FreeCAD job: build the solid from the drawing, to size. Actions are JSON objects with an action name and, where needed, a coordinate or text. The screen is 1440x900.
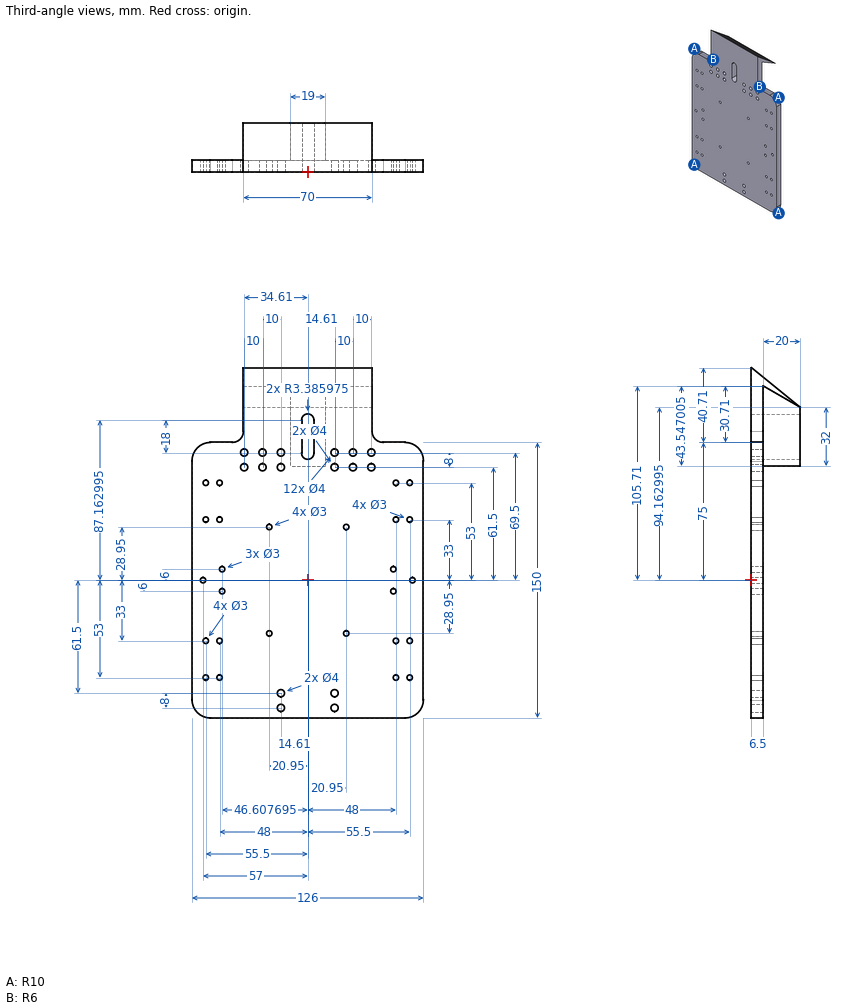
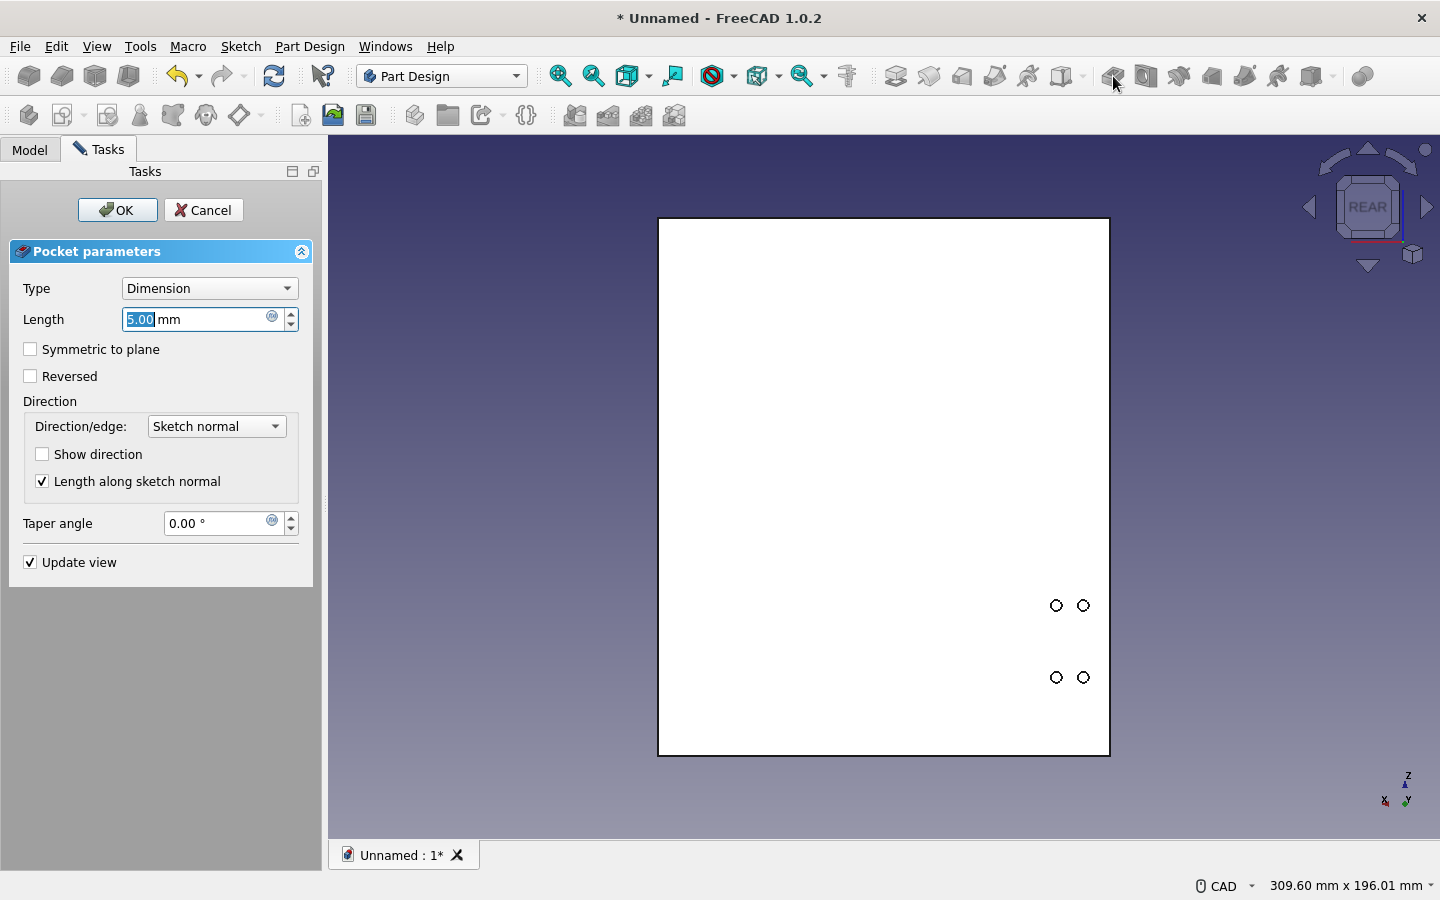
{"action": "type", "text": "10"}
{"action": "key", "text": "Tab"}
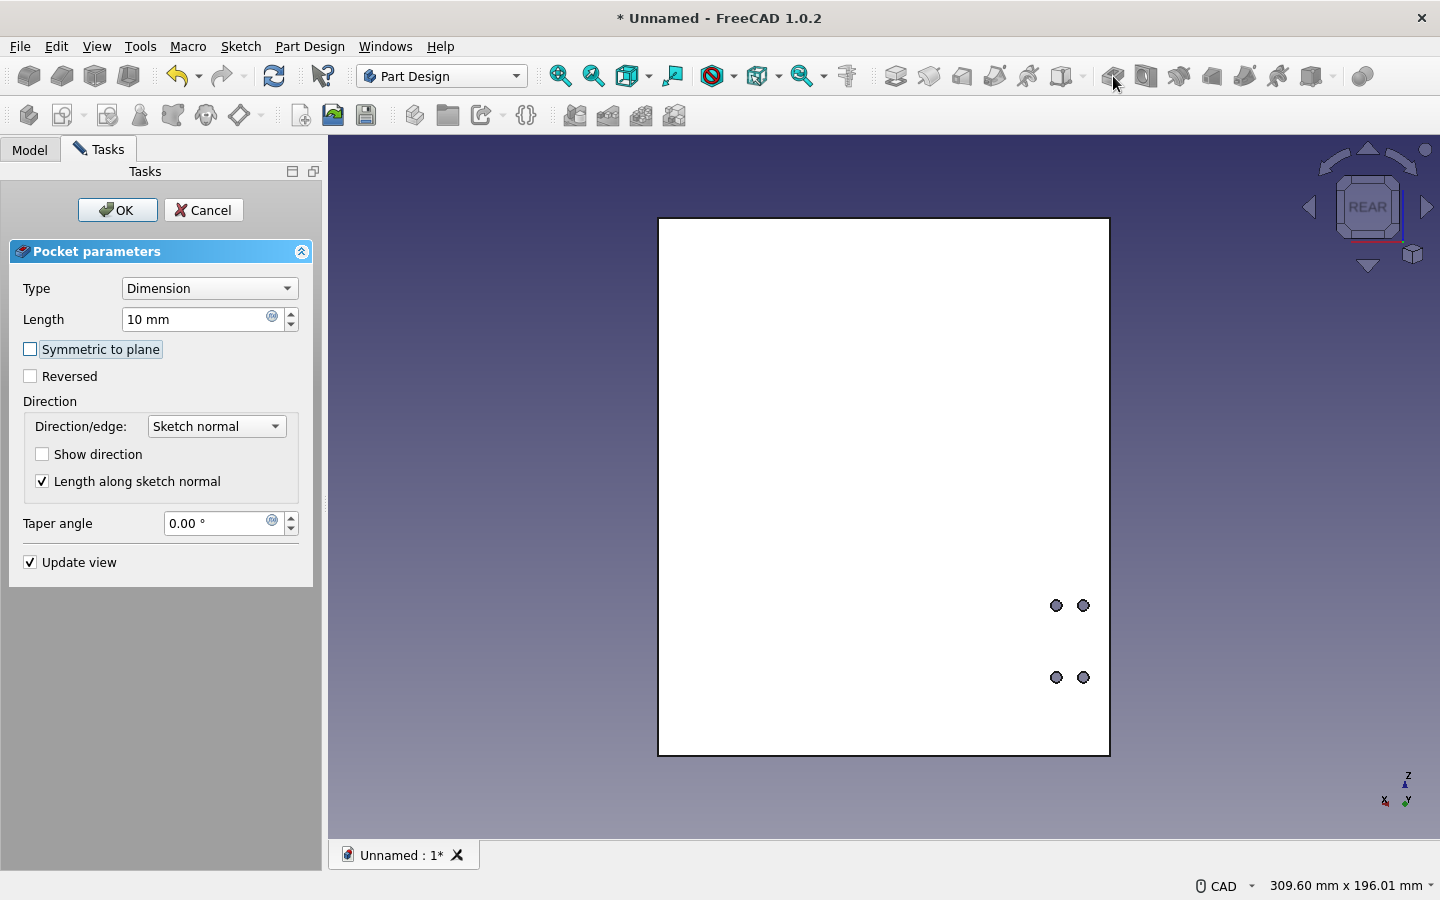
{"action": "left_click", "coordinate": [118, 210]}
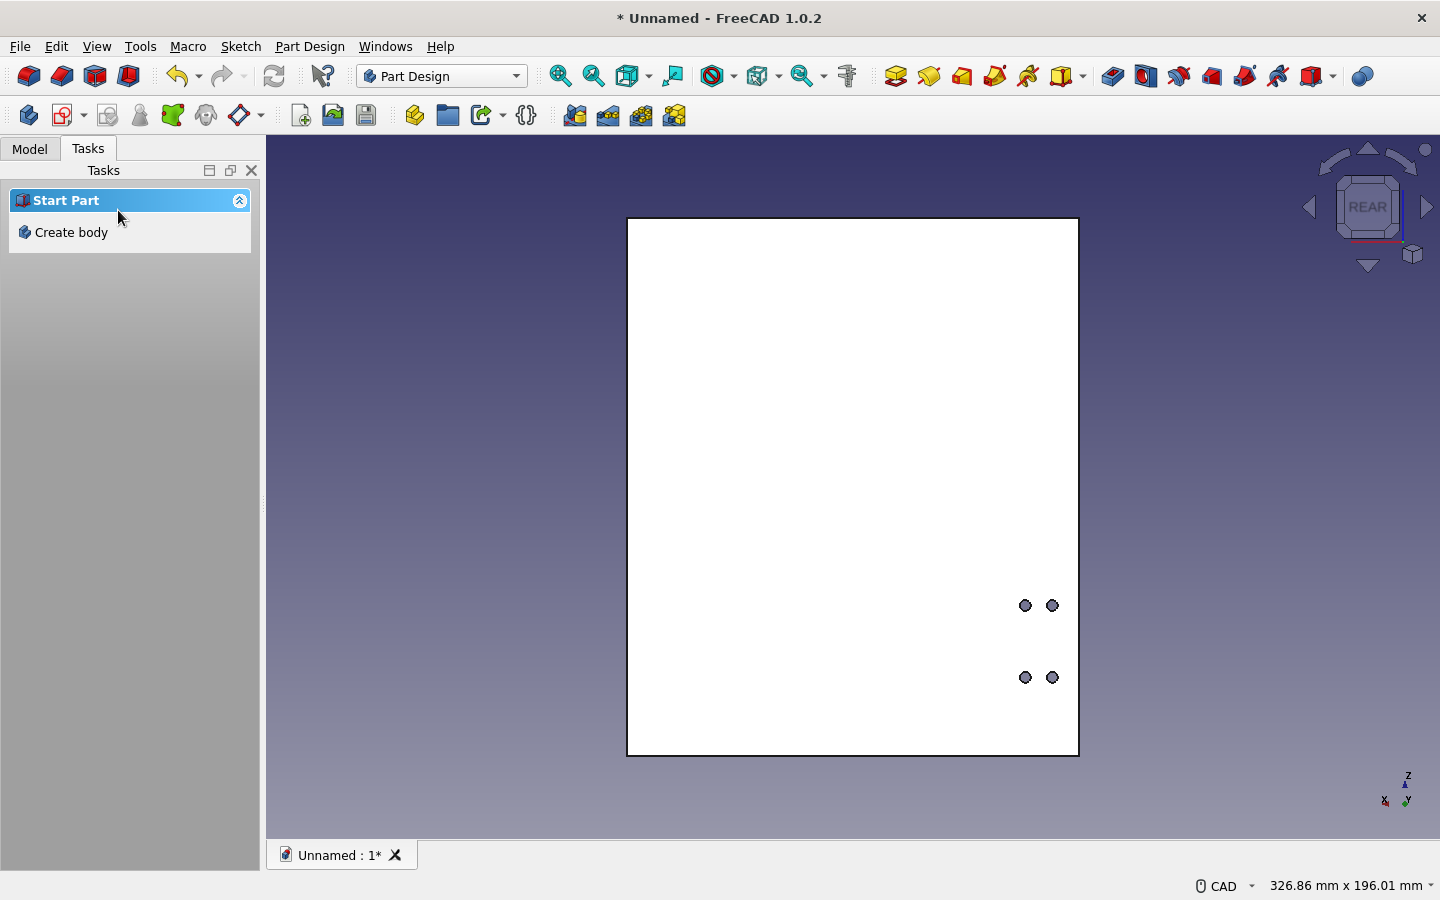
{"action": "left_click", "coordinate": [30, 148]}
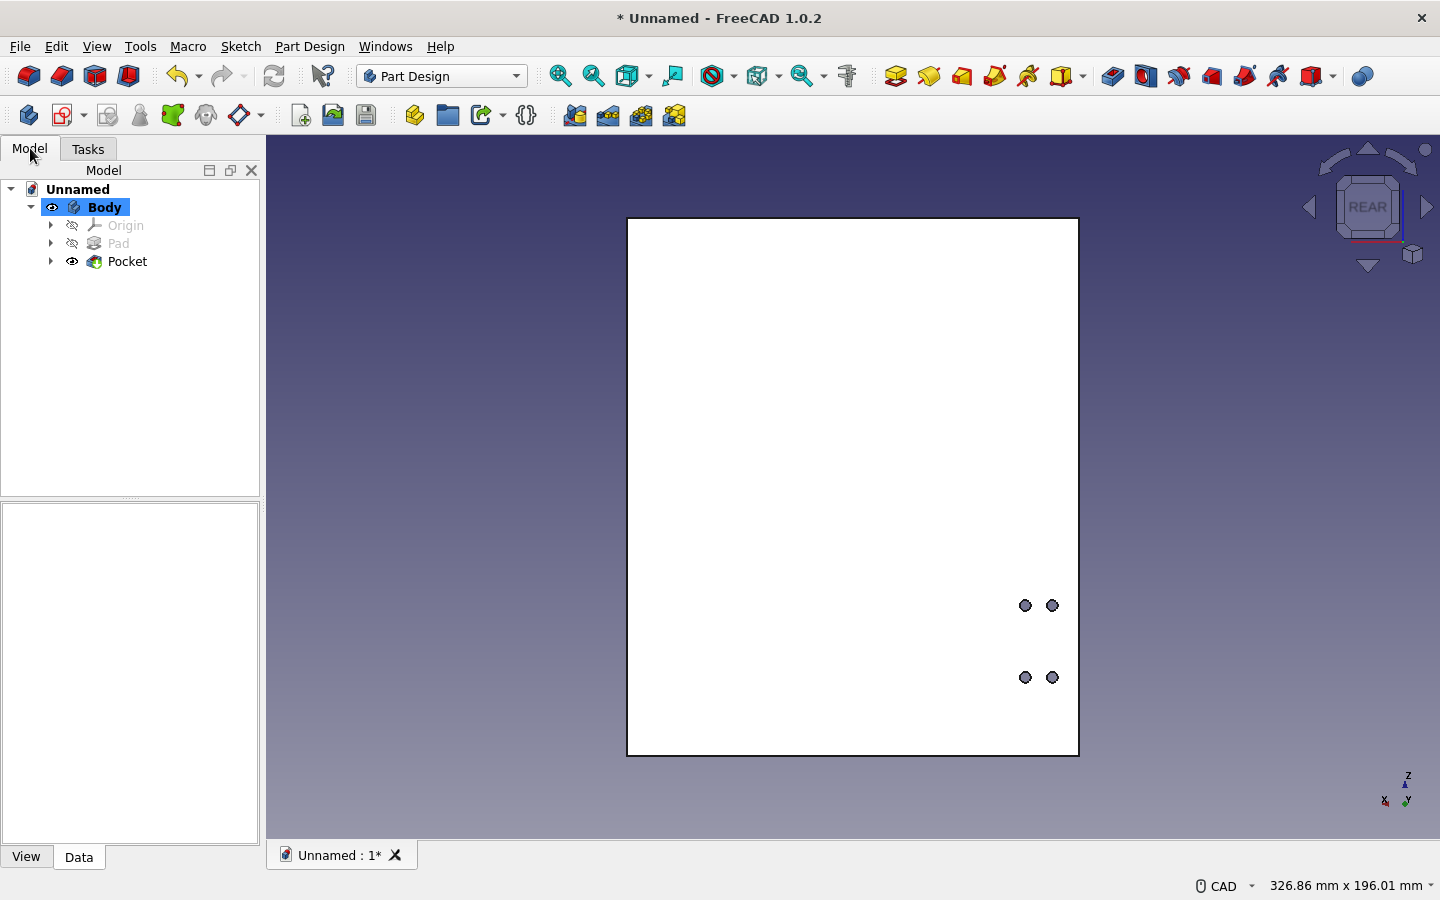
{"action": "left_click", "coordinate": [117, 261]}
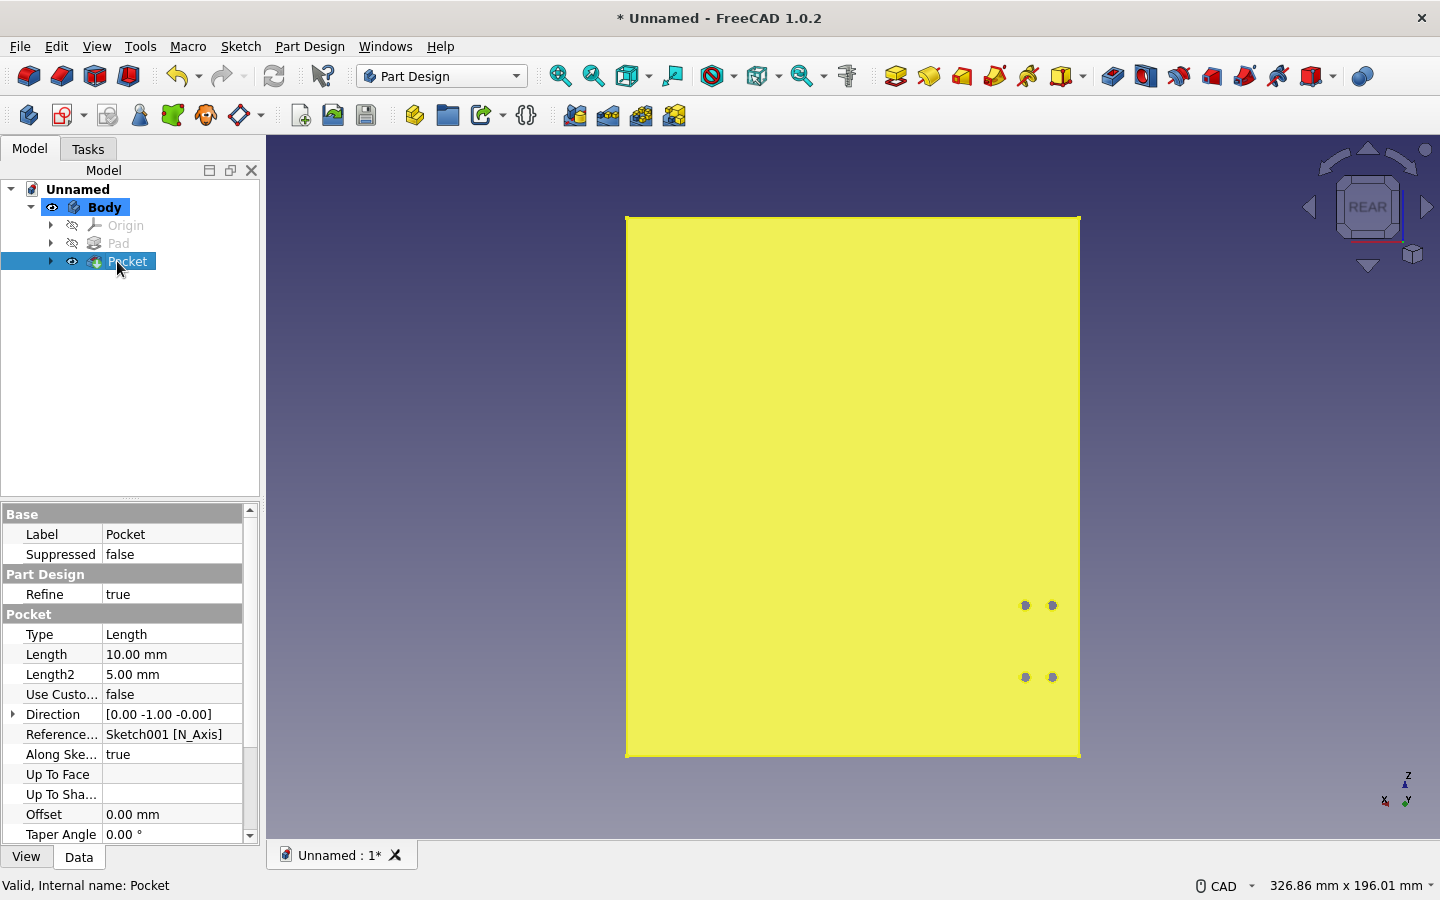
{"action": "left_click", "coordinate": [575, 116]}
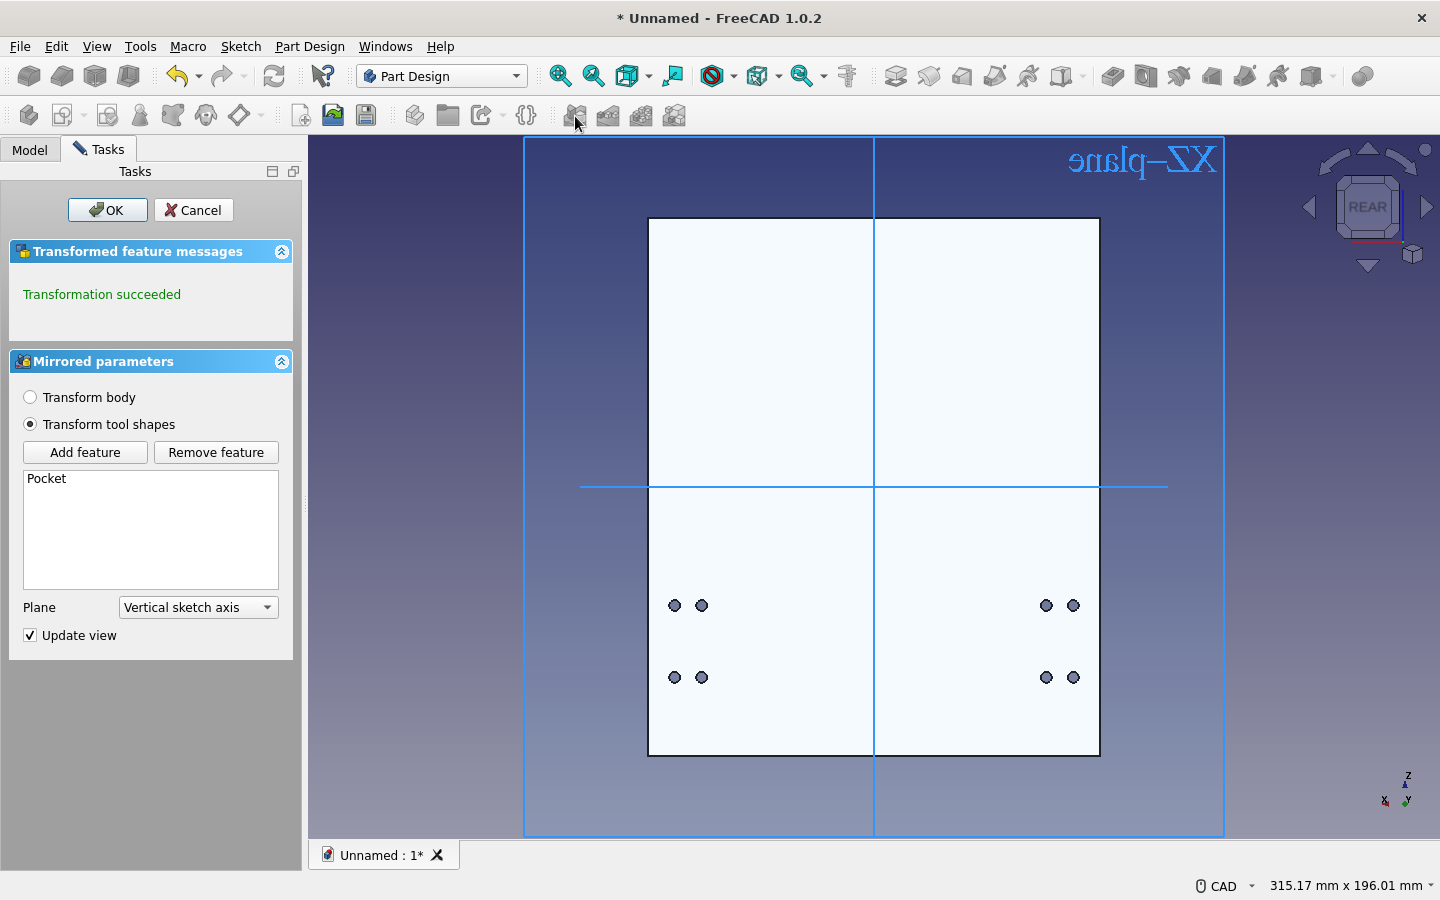
{"action": "left_click", "coordinate": [199, 608]}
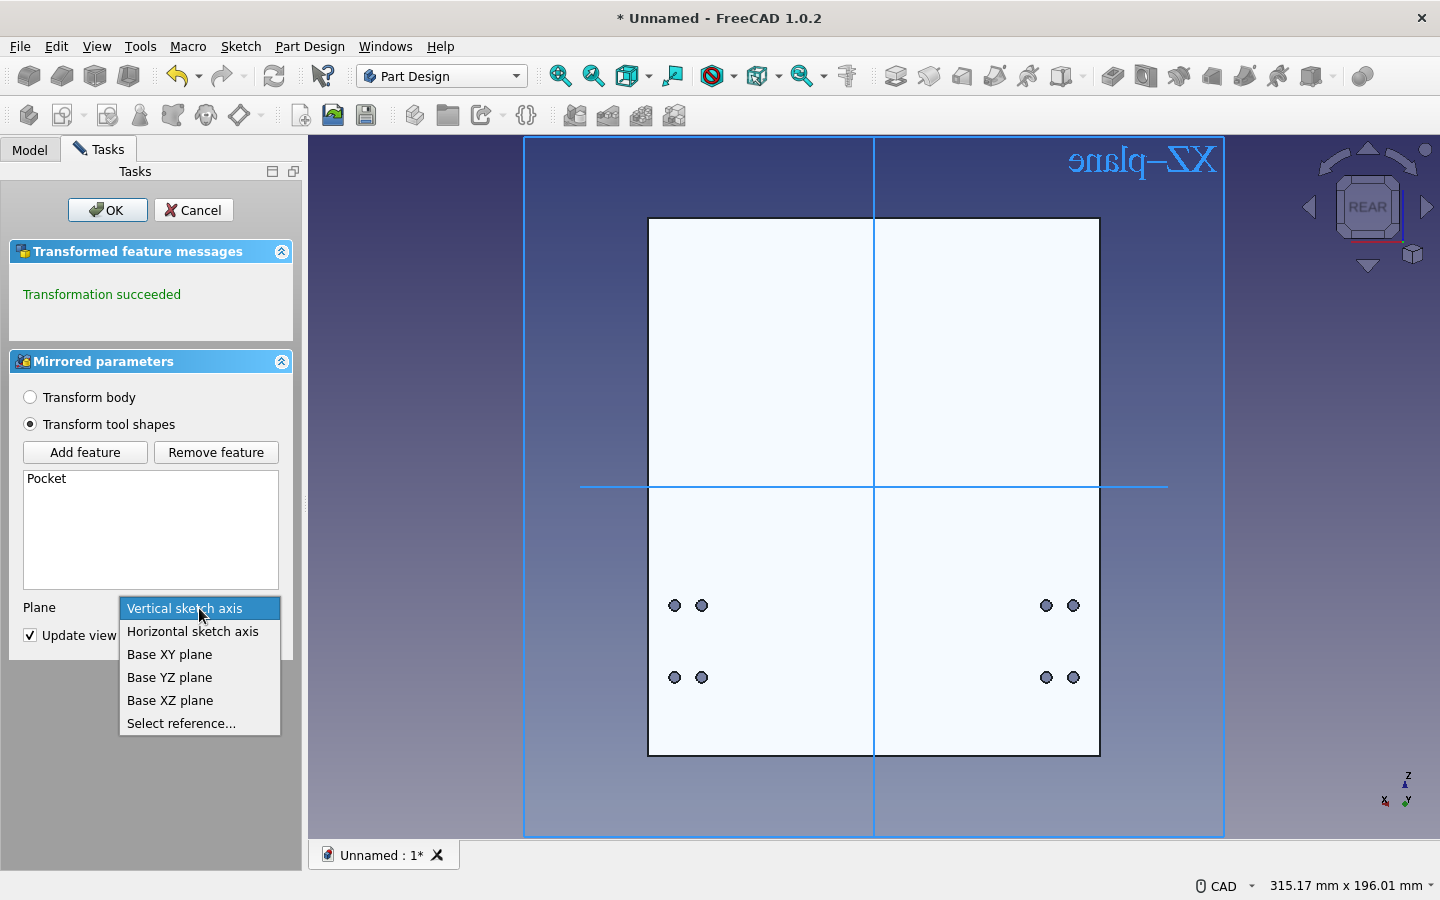
{"action": "left_click", "coordinate": [198, 678]}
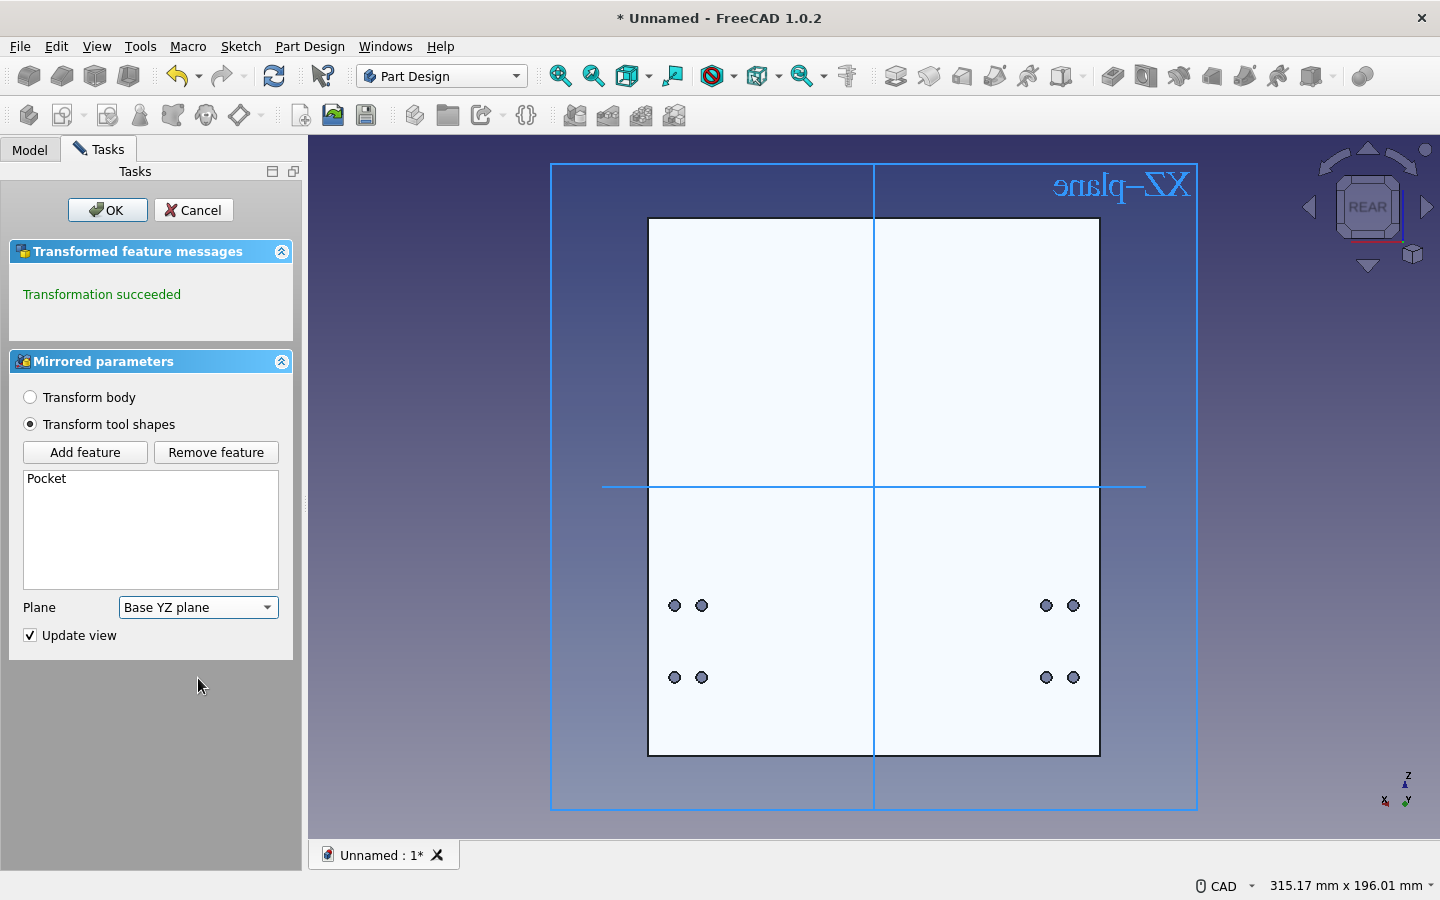
{"action": "left_click", "coordinate": [108, 210]}